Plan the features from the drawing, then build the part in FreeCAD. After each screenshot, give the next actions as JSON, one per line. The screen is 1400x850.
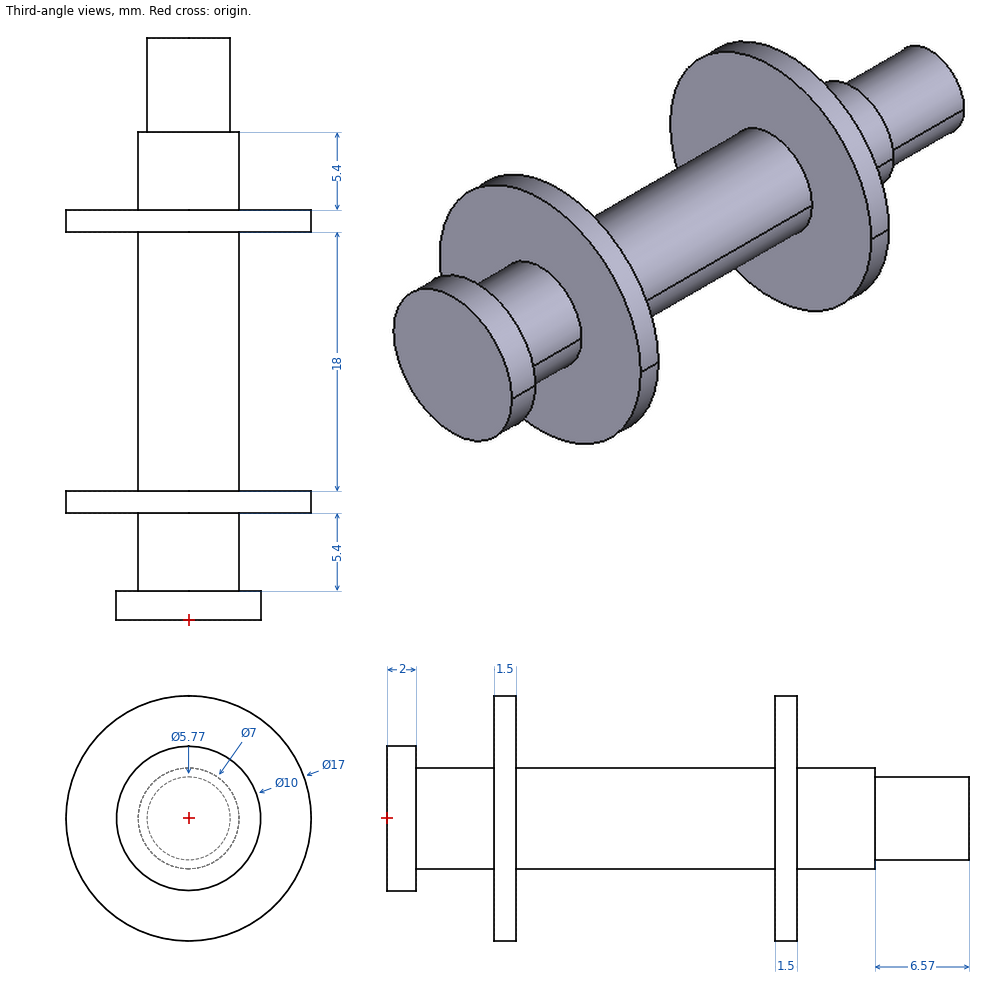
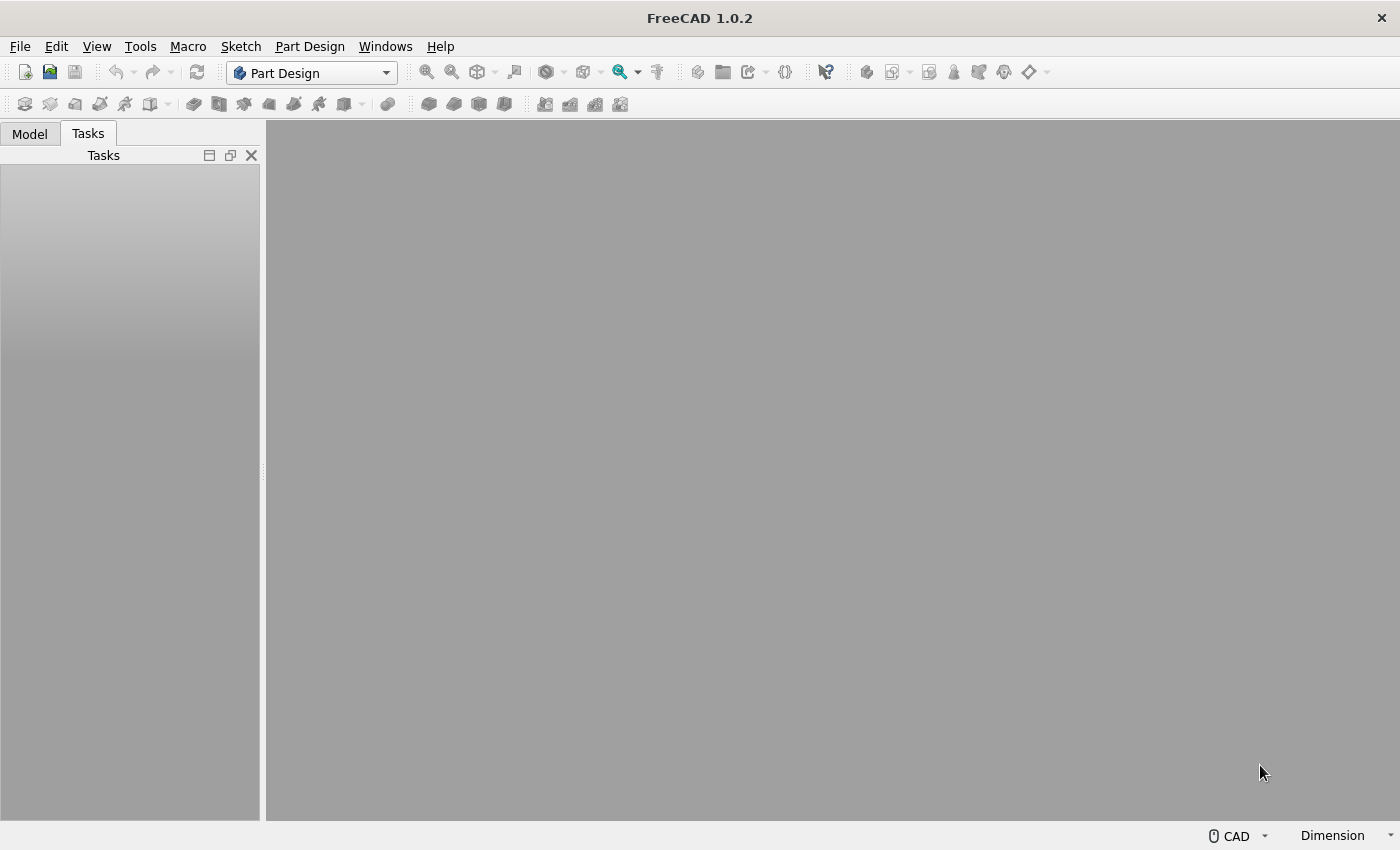
{"action": "left_click", "coordinate": [25, 72]}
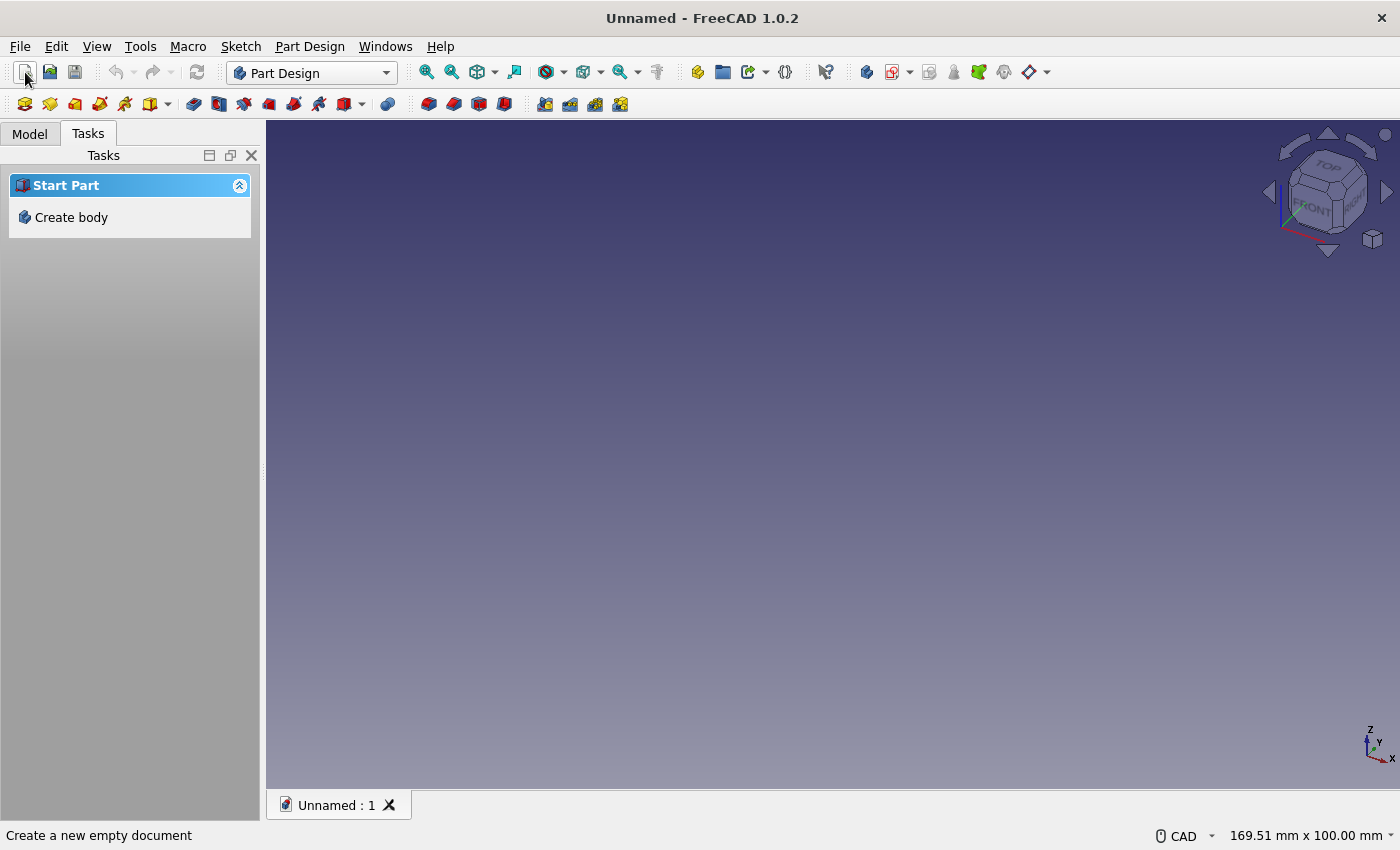
{"action": "left_click", "coordinate": [892, 72]}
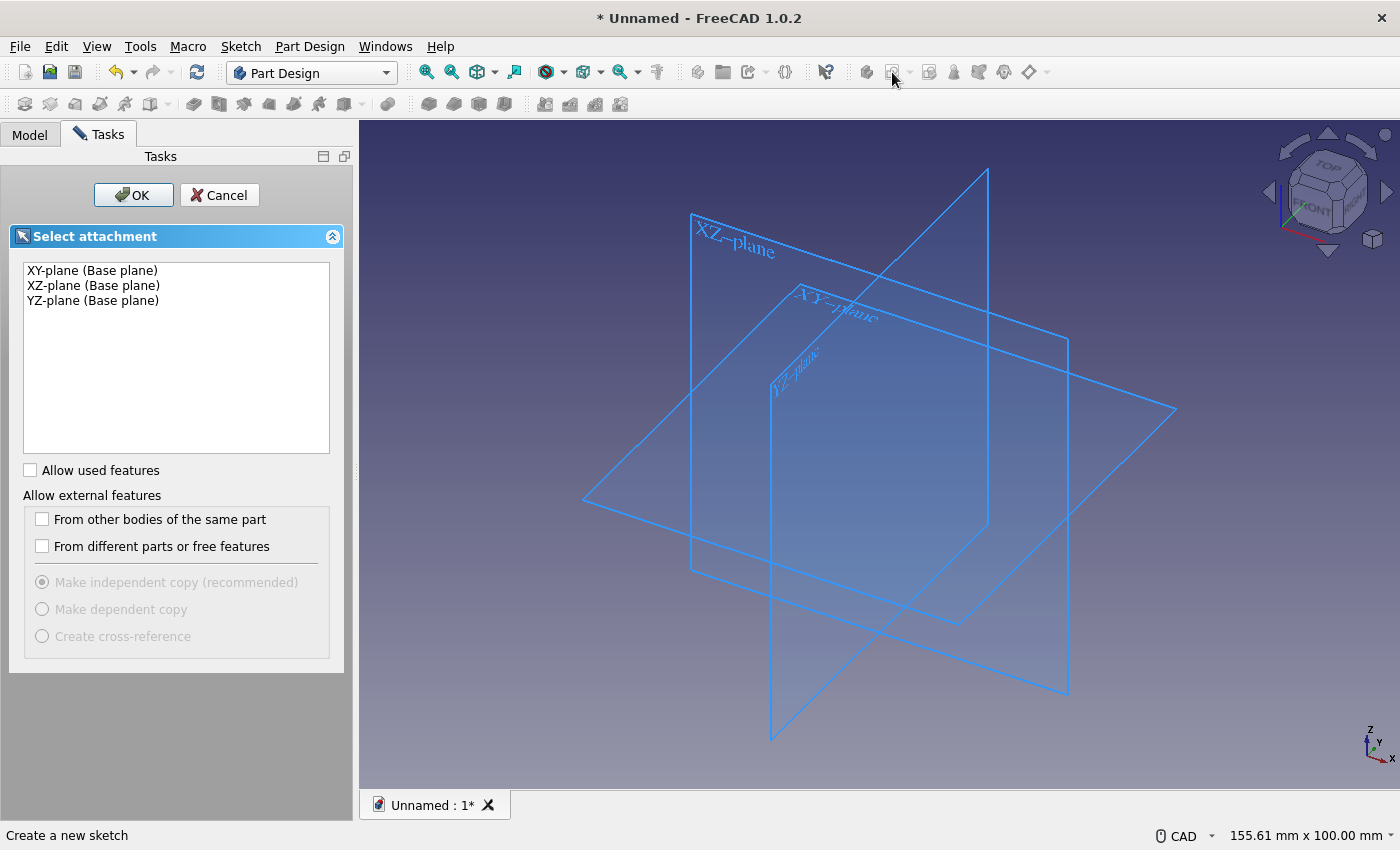
{"action": "left_click", "coordinate": [84, 286]}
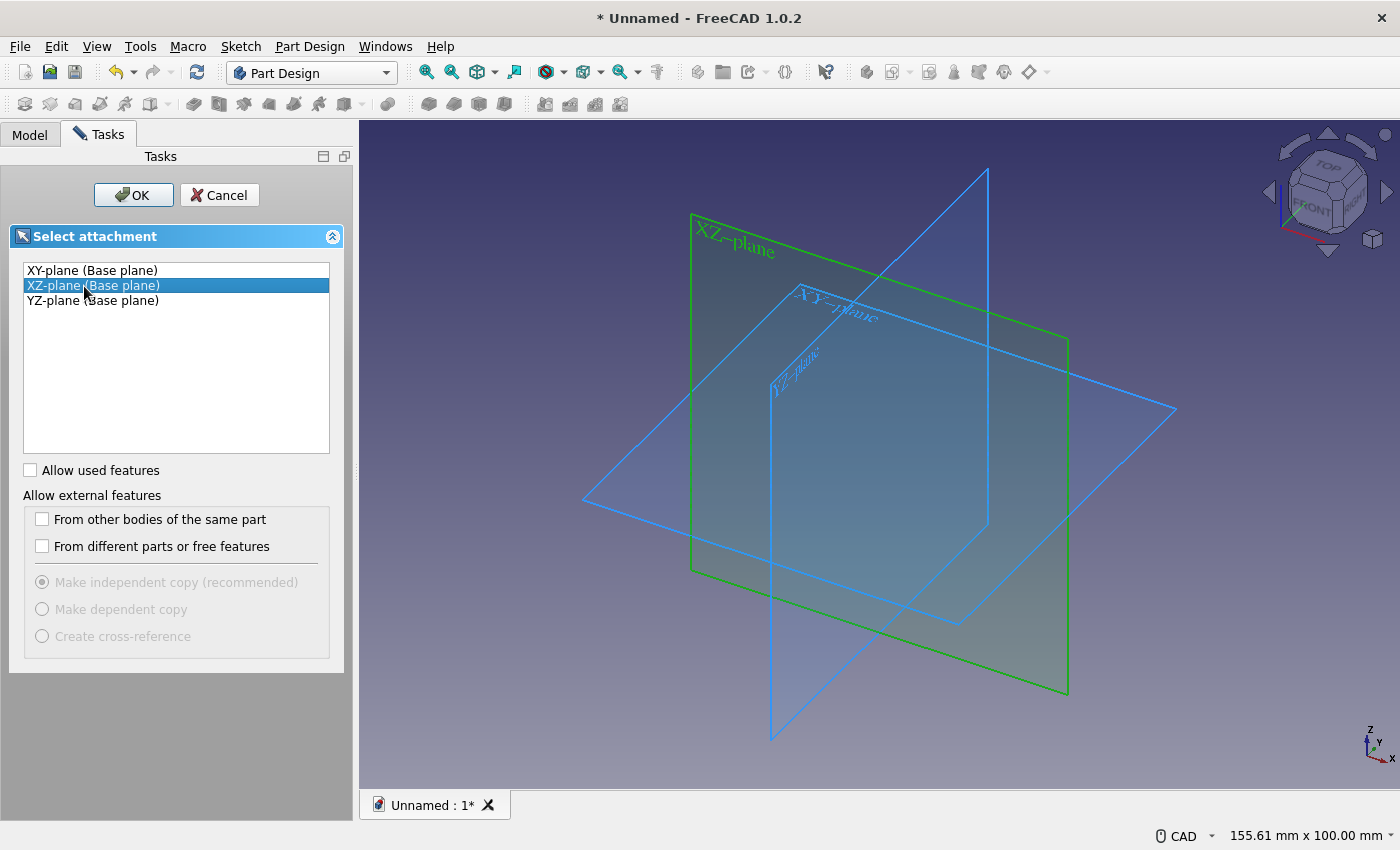
{"action": "left_click", "coordinate": [134, 195]}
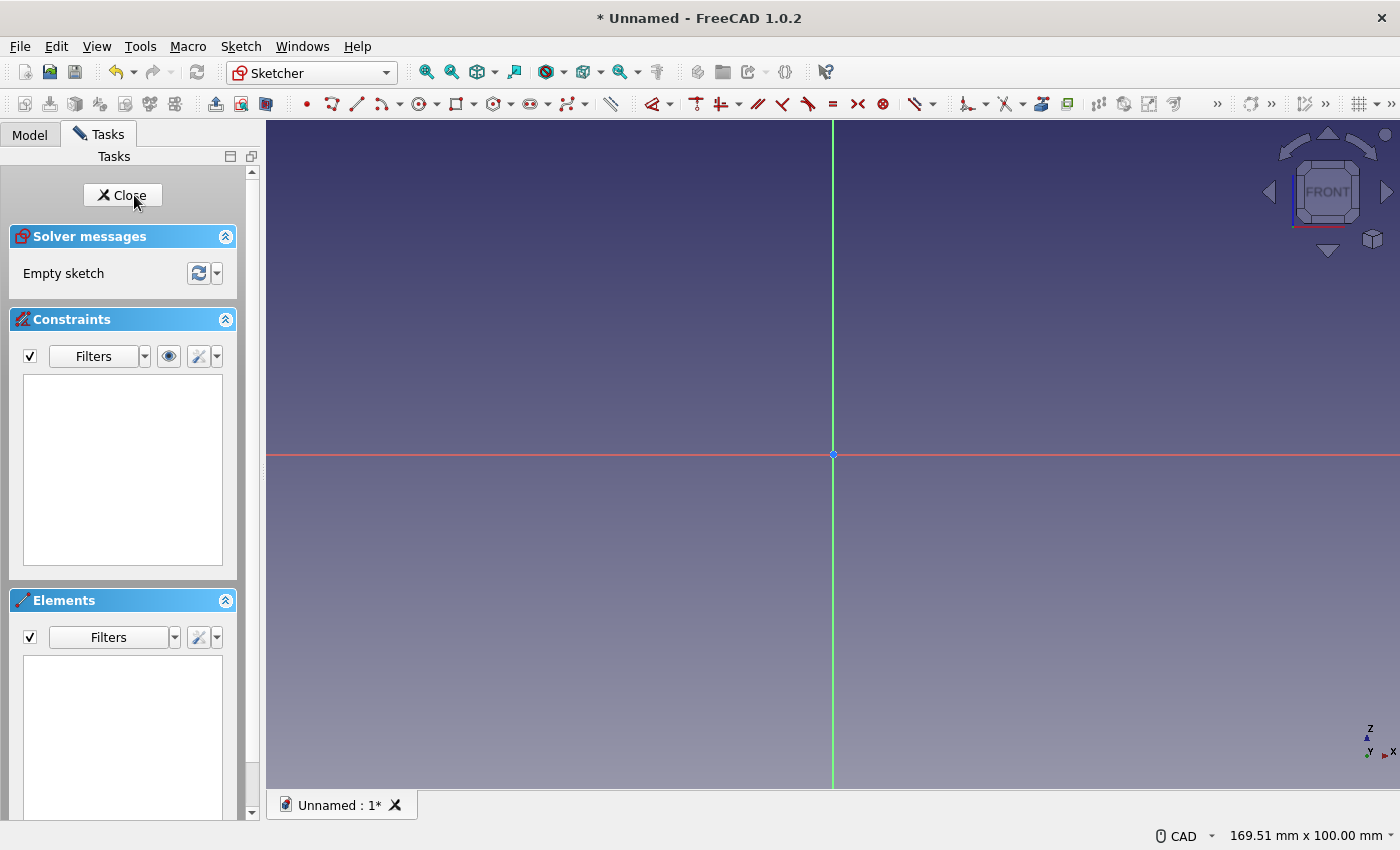
{"action": "scroll", "coordinate": [847, 455], "scroll_direction": "up", "scroll_amount": 9}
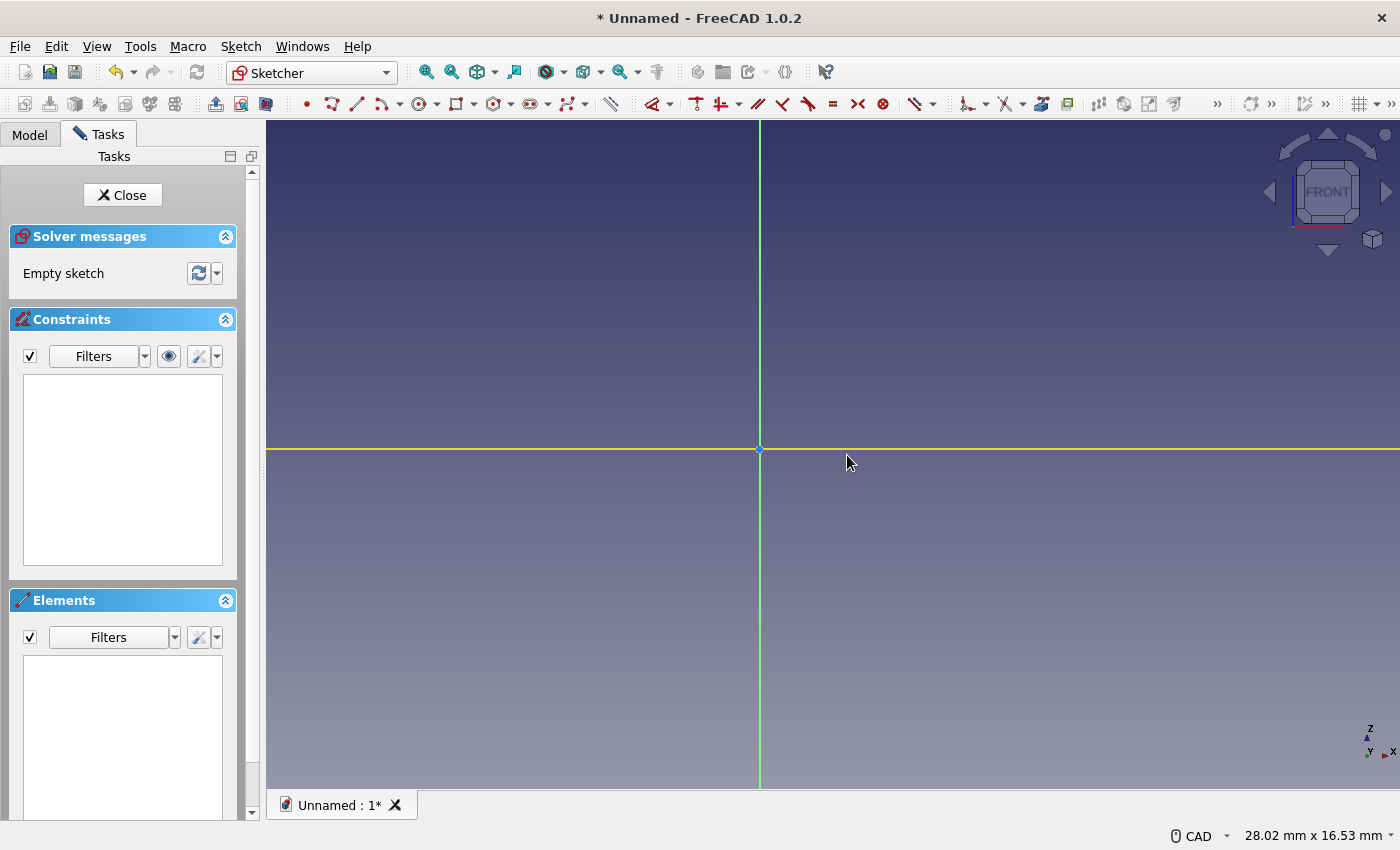
{"action": "left_click", "coordinate": [418, 104]}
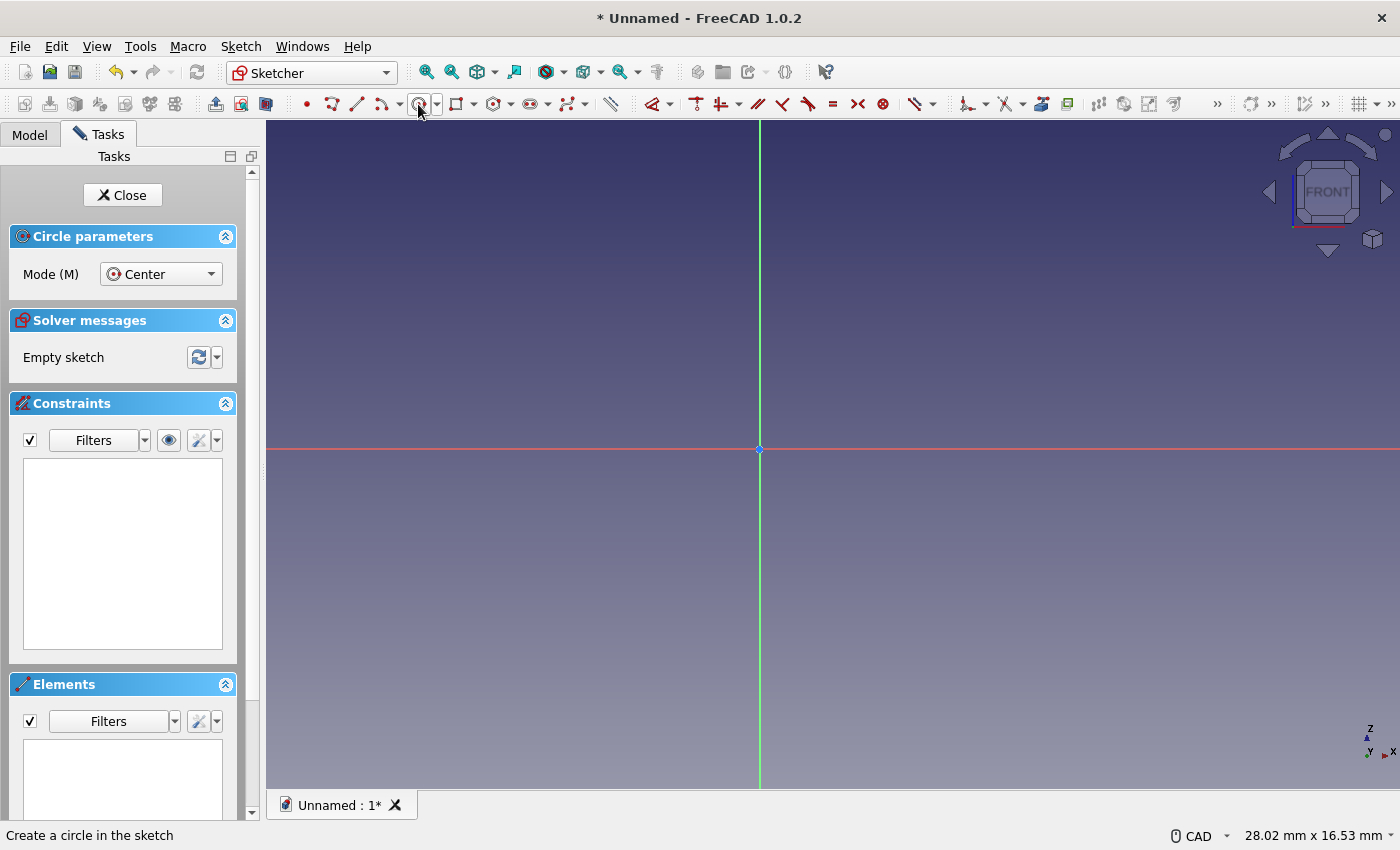
{"action": "left_click", "coordinate": [760, 449]}
{"action": "left_click", "coordinate": [903, 306]}
{"action": "key", "text": "Escape"}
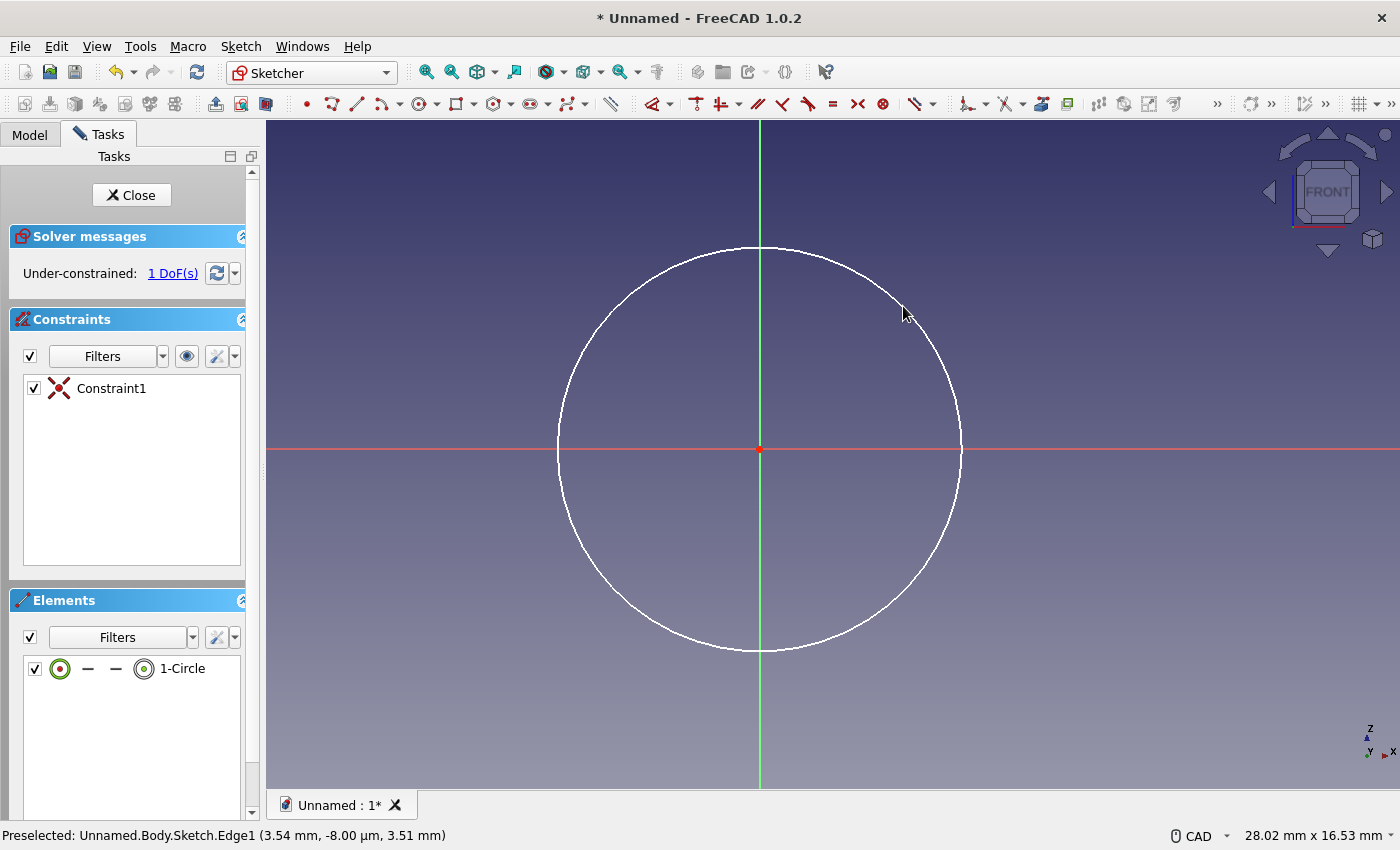
{"action": "left_click", "coordinate": [652, 104]}